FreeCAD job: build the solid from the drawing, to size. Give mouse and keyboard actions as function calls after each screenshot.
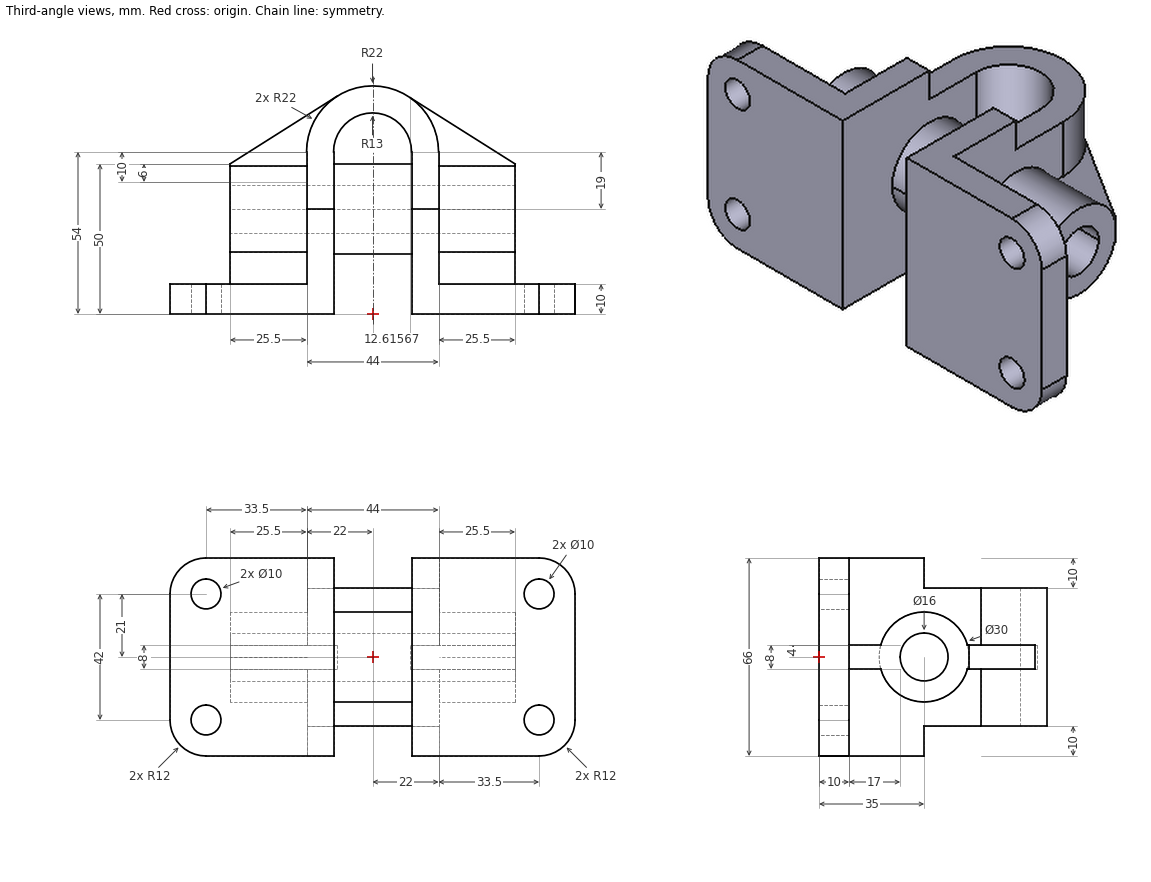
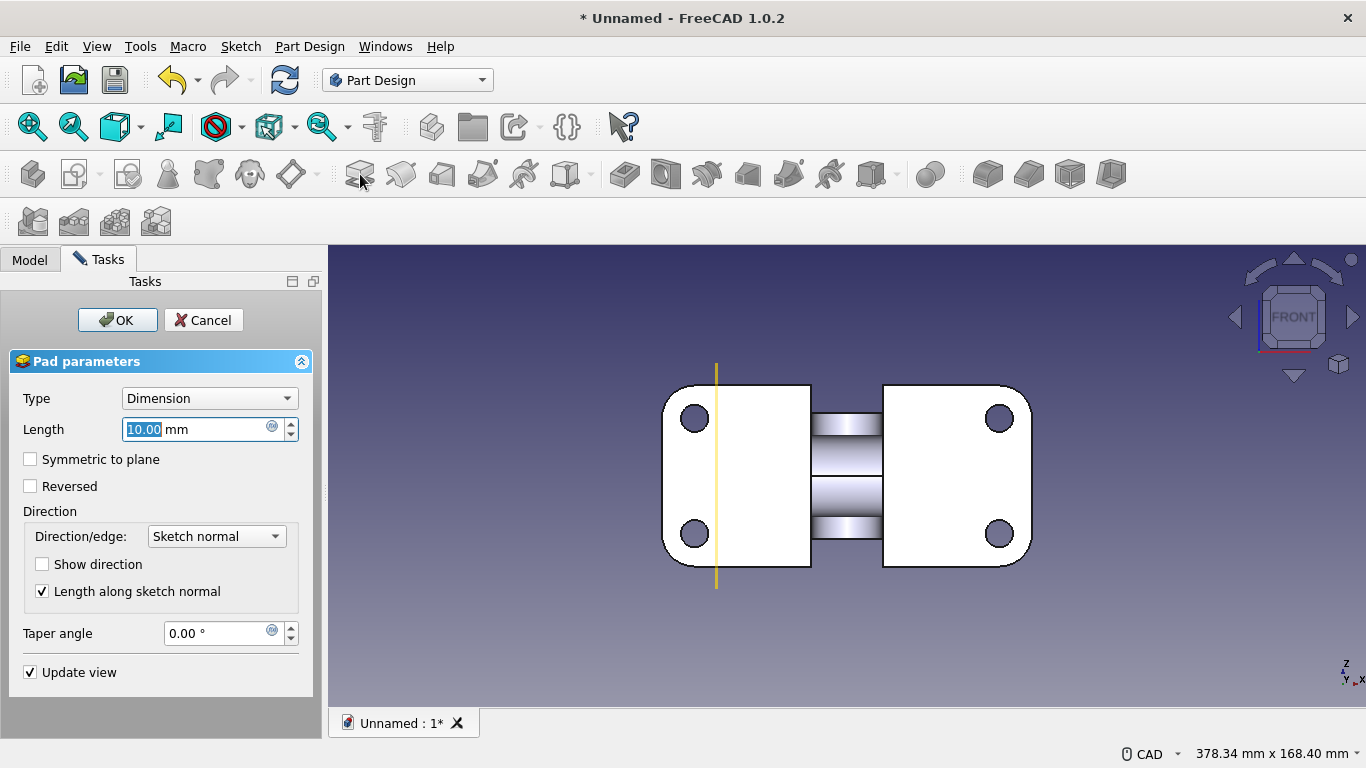
text(25.5)
key(Tab)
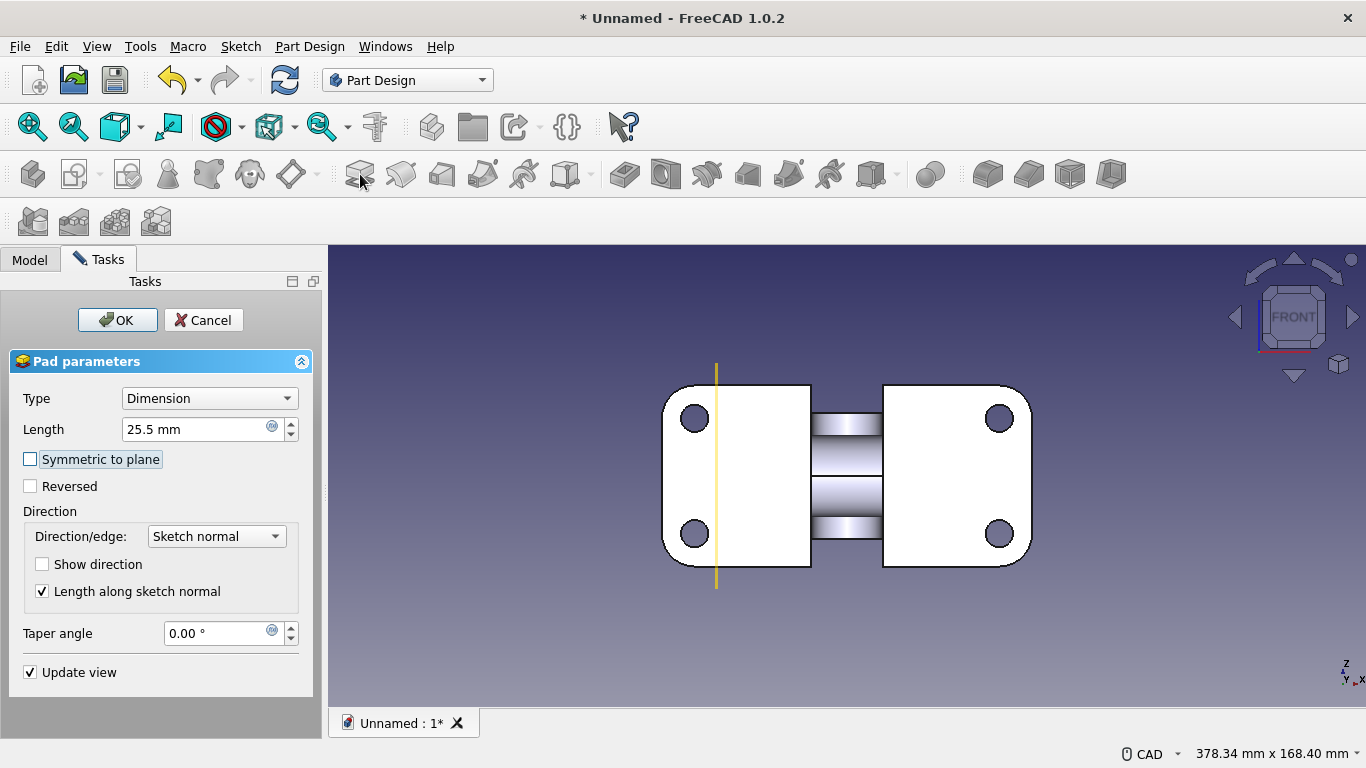
click(118, 320)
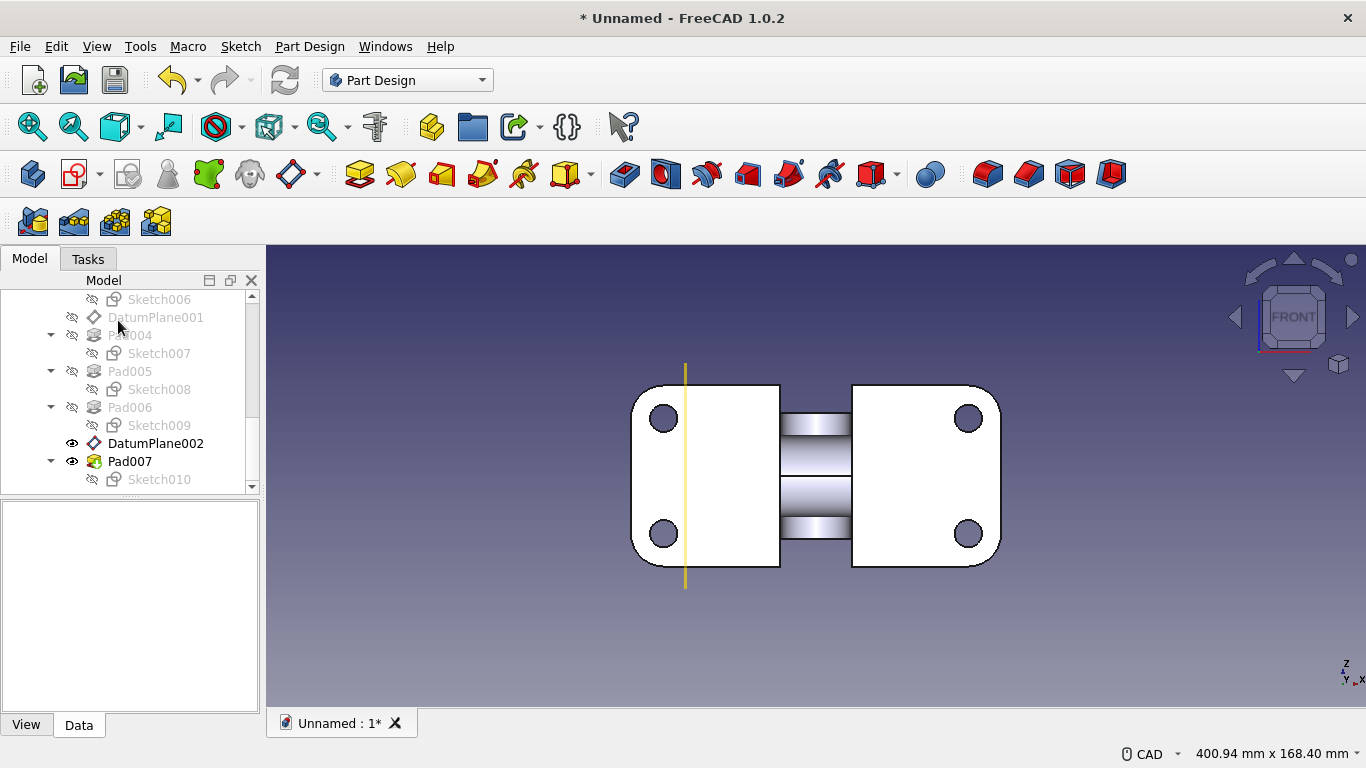
click(117, 443)
key(space)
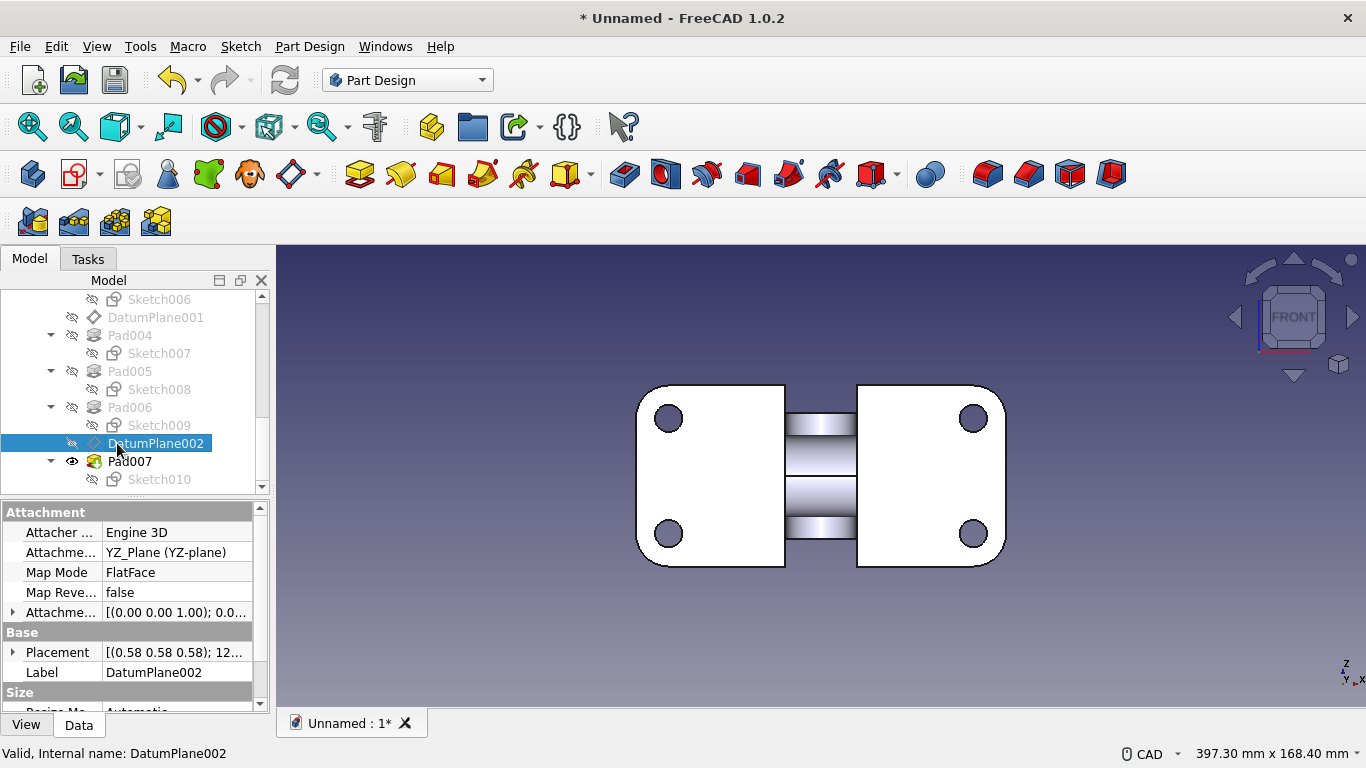
click(33, 128)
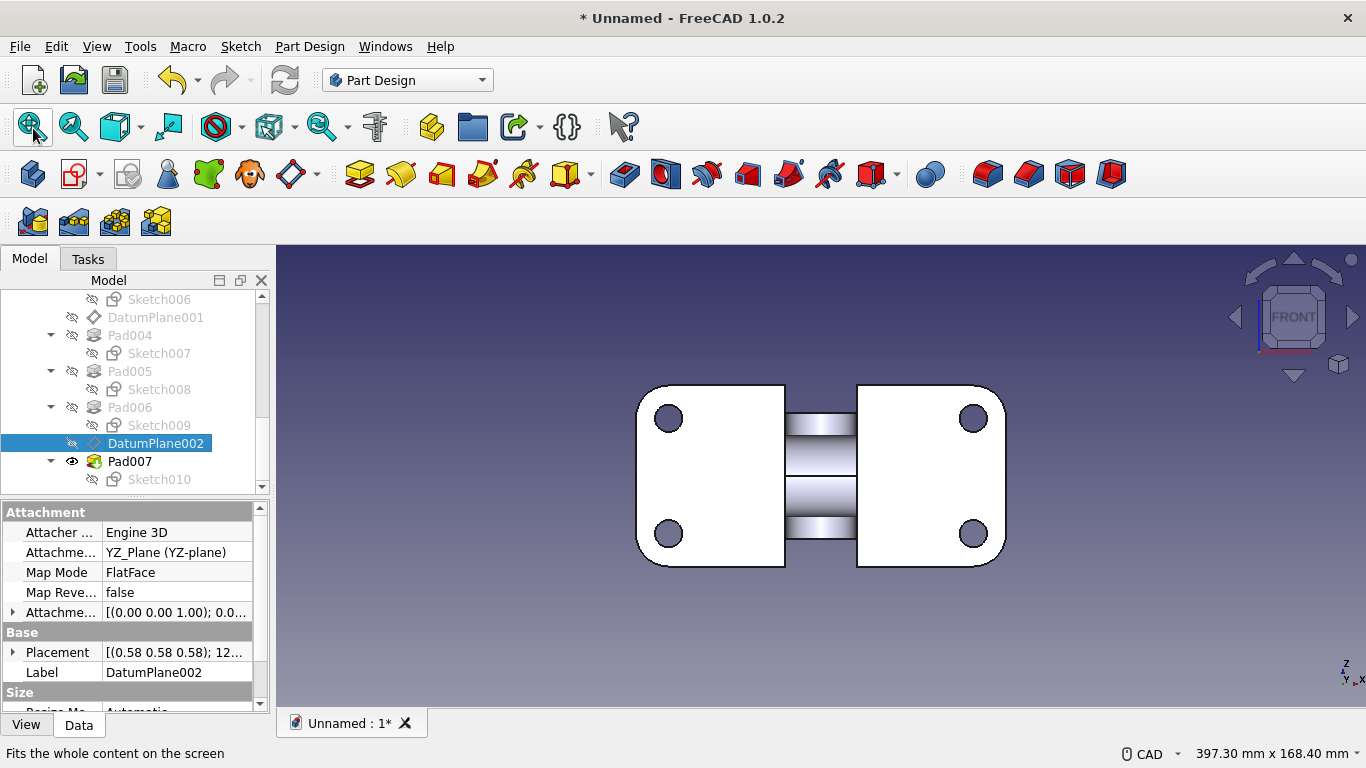
click(316, 667)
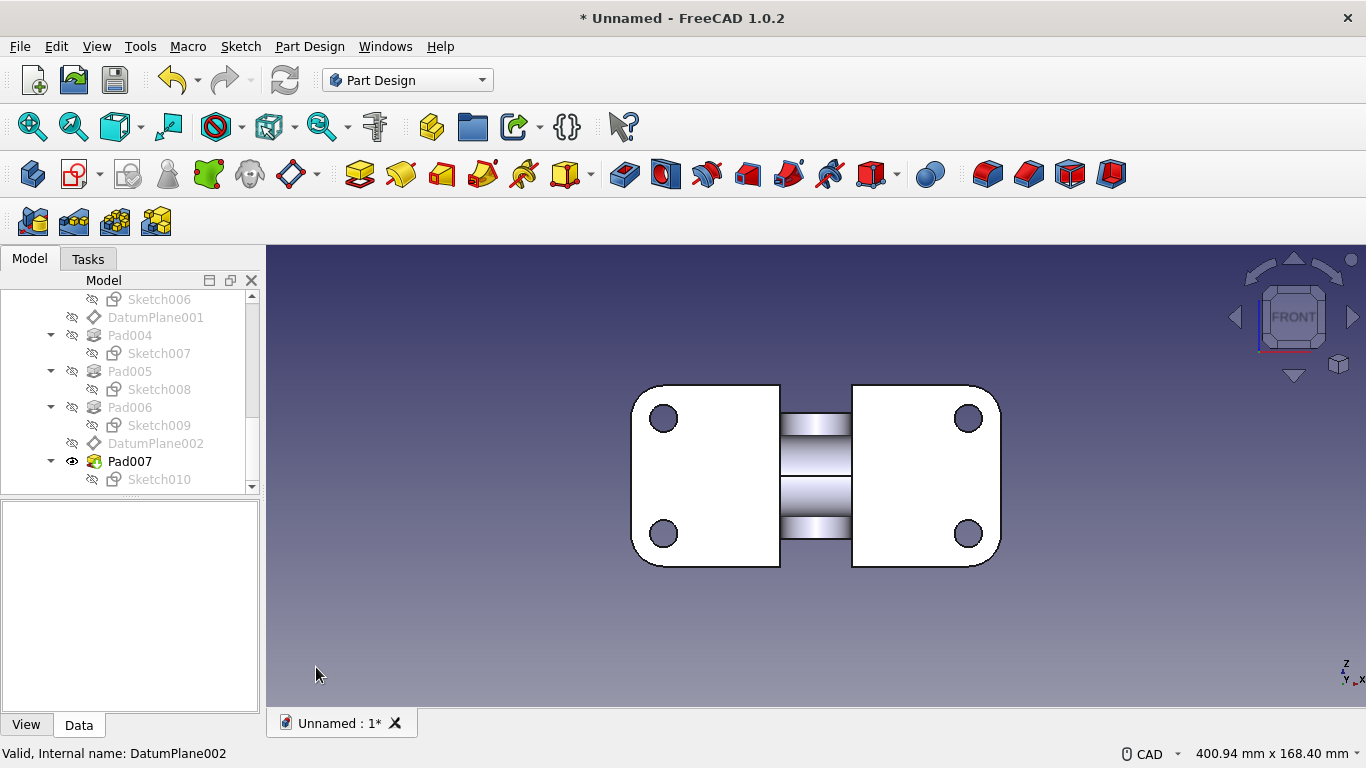
click(74, 174)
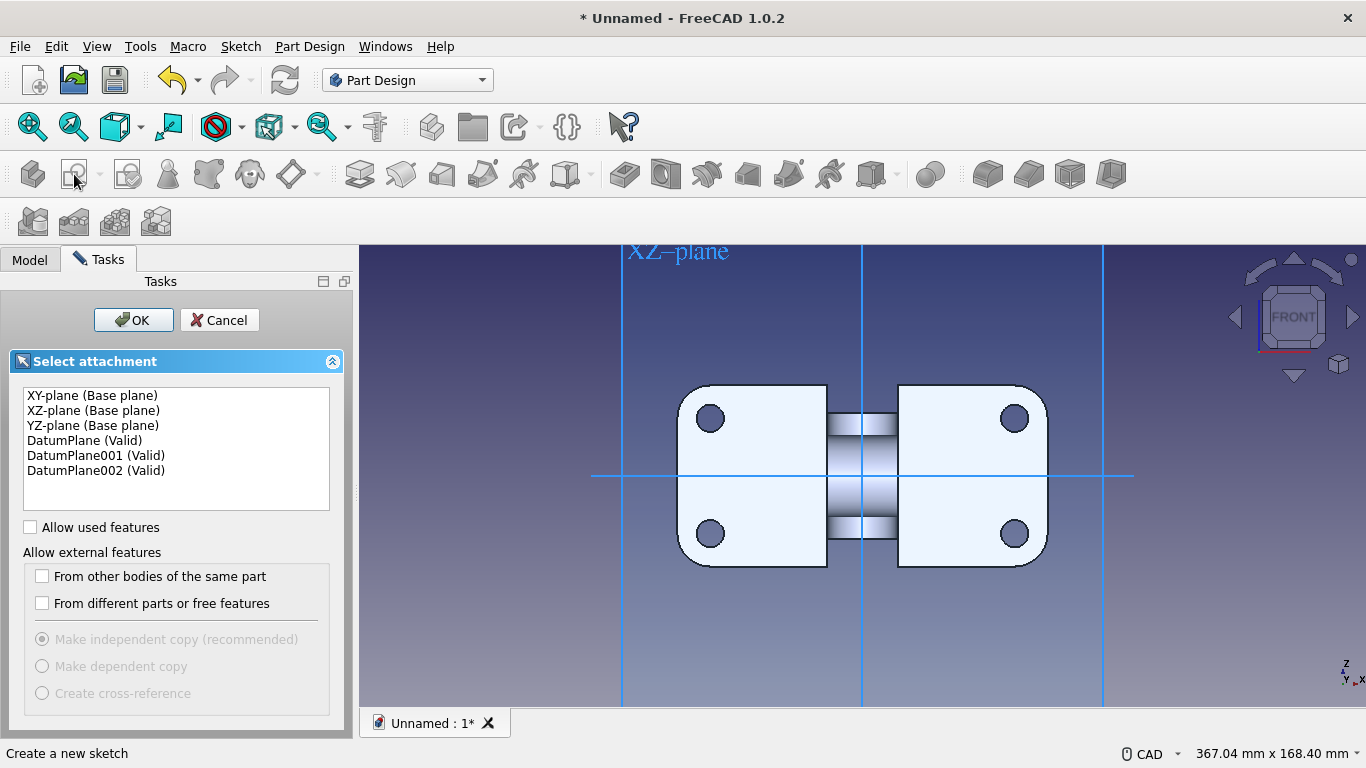
click(84, 396)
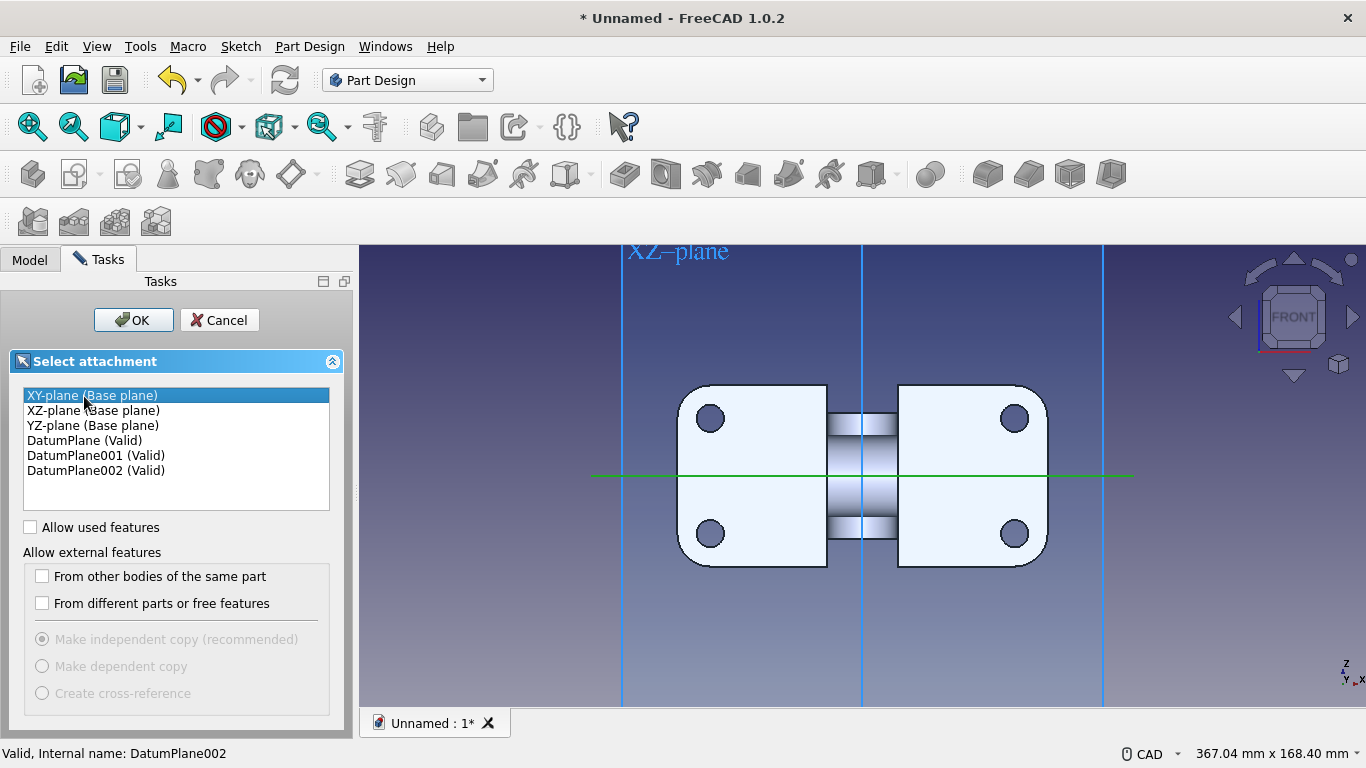
click(134, 320)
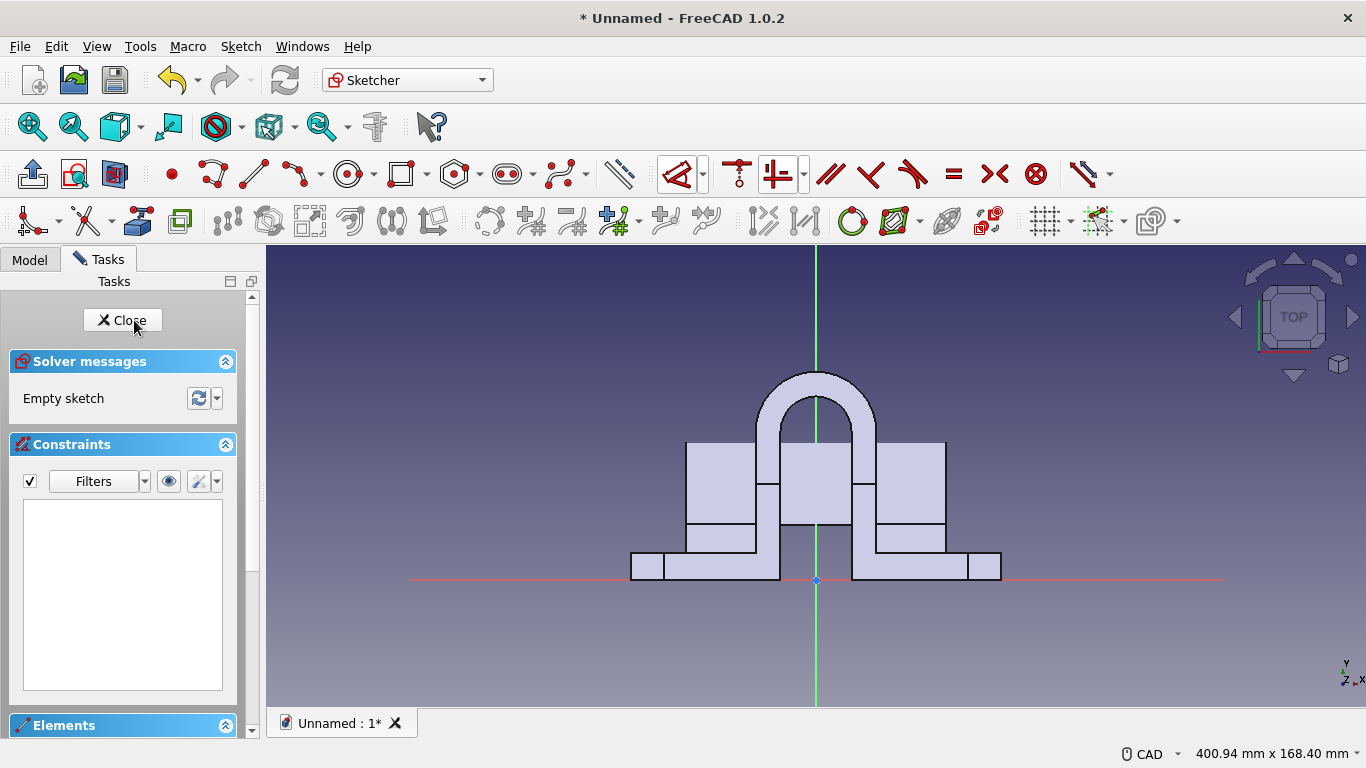
click(115, 174)